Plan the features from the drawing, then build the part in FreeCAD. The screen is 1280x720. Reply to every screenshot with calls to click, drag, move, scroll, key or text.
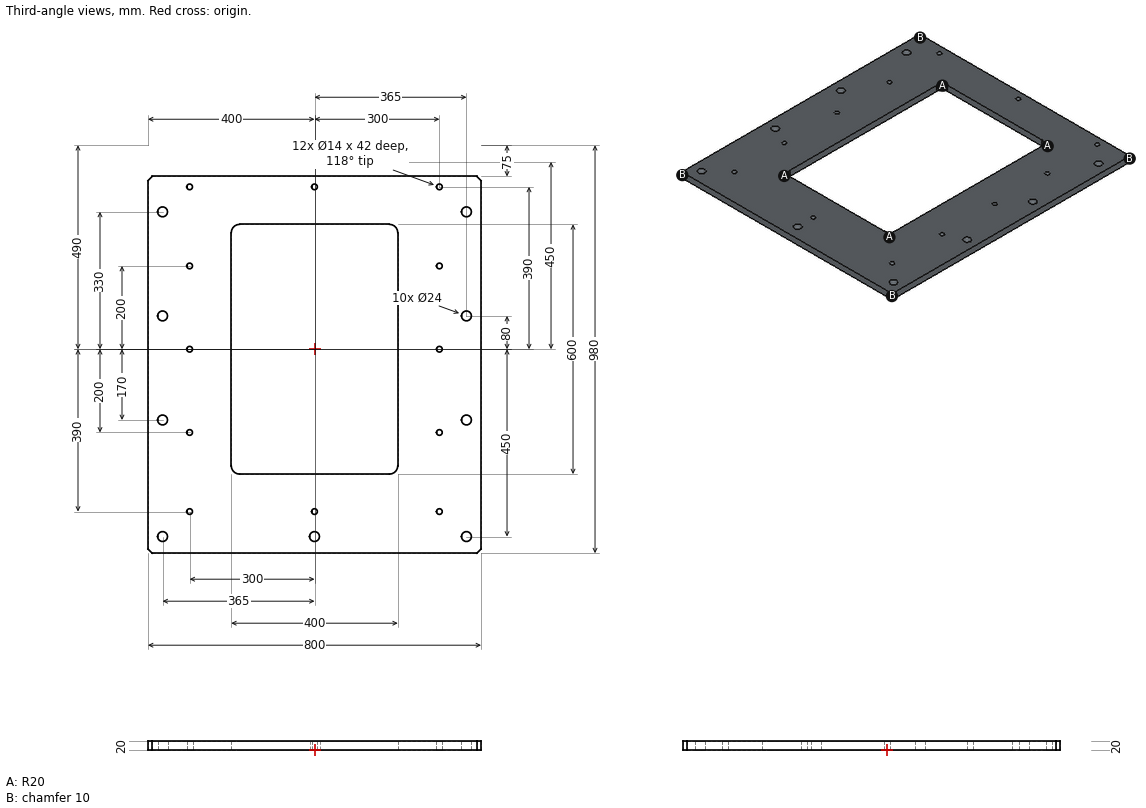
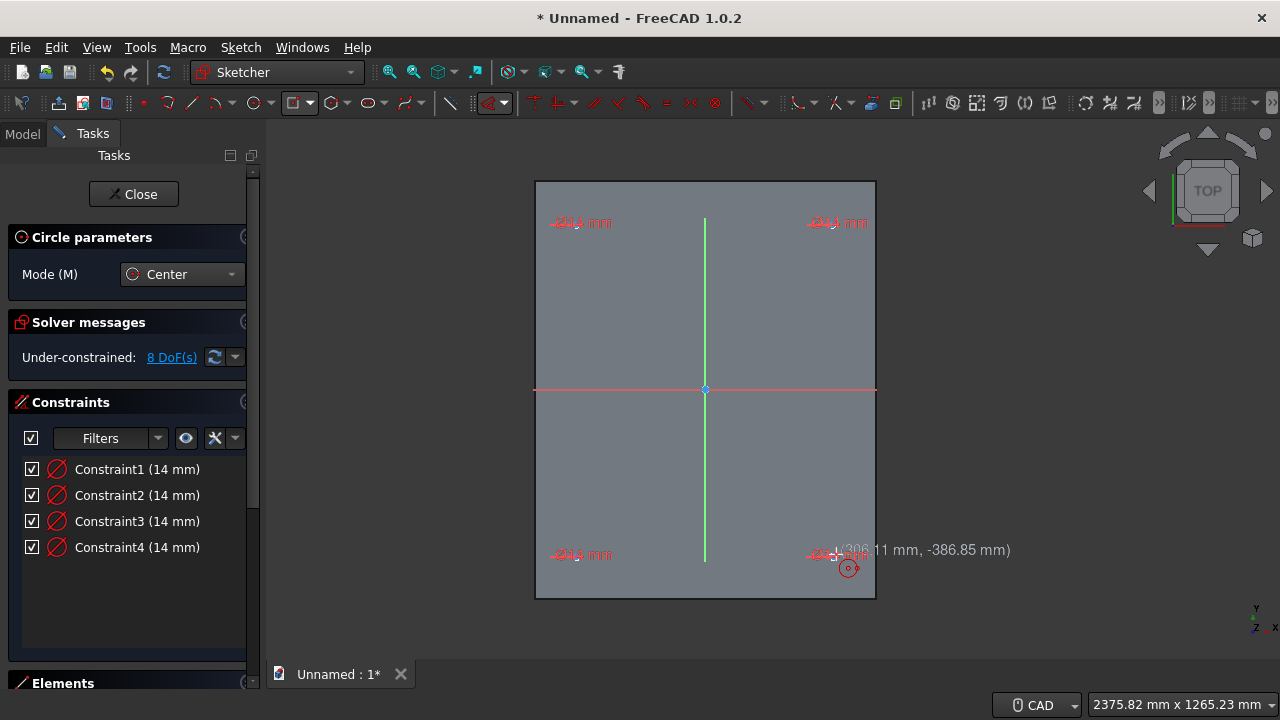
scroll(577, 390, up, 11)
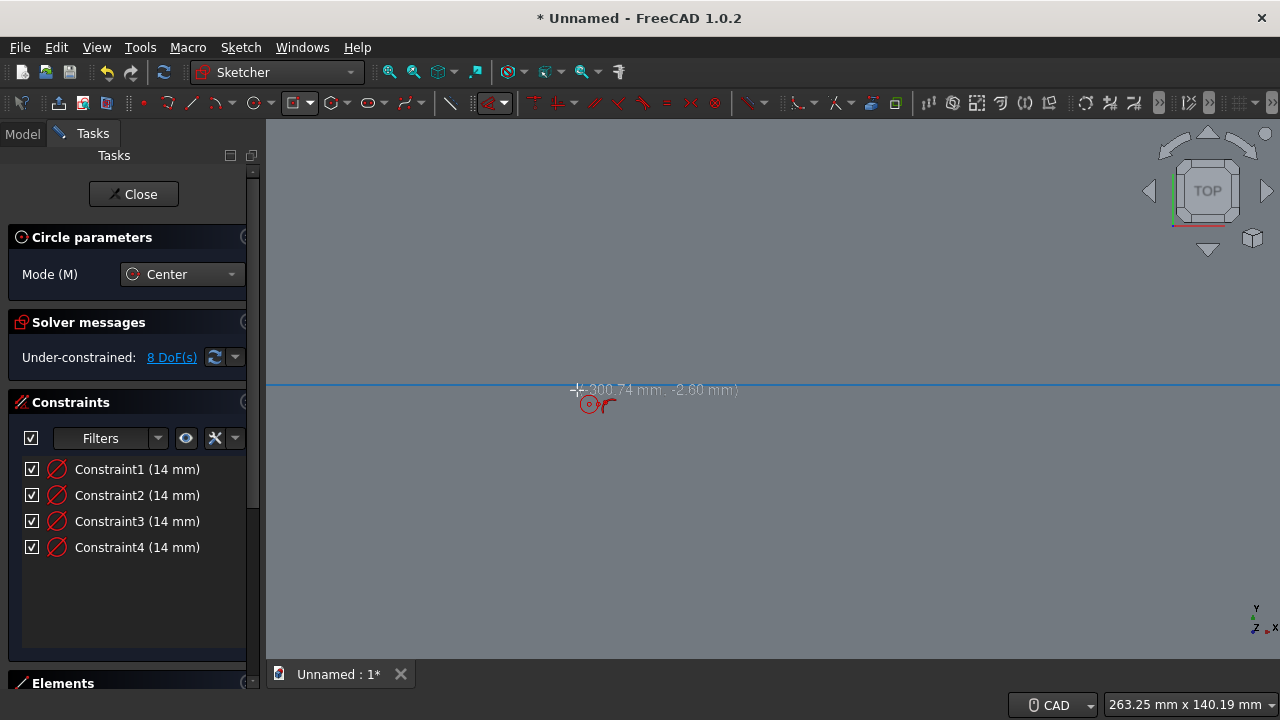
scroll(576, 390, down, 11)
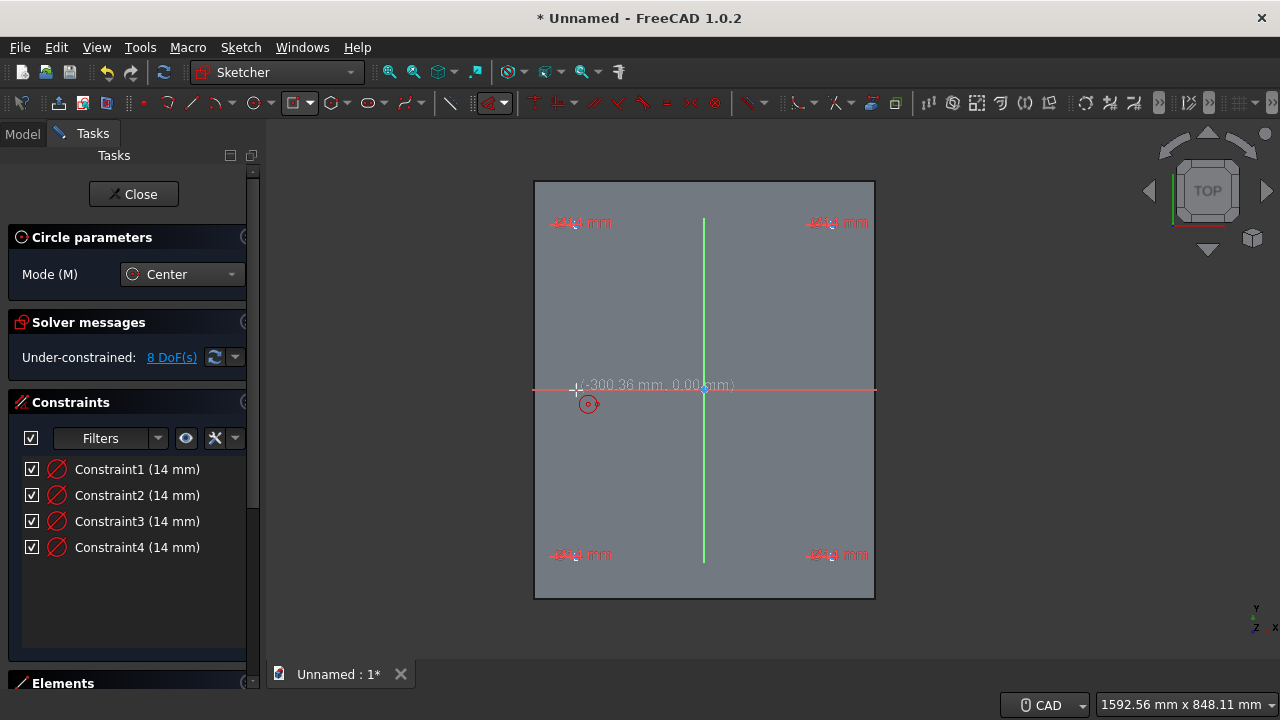
click(576, 390)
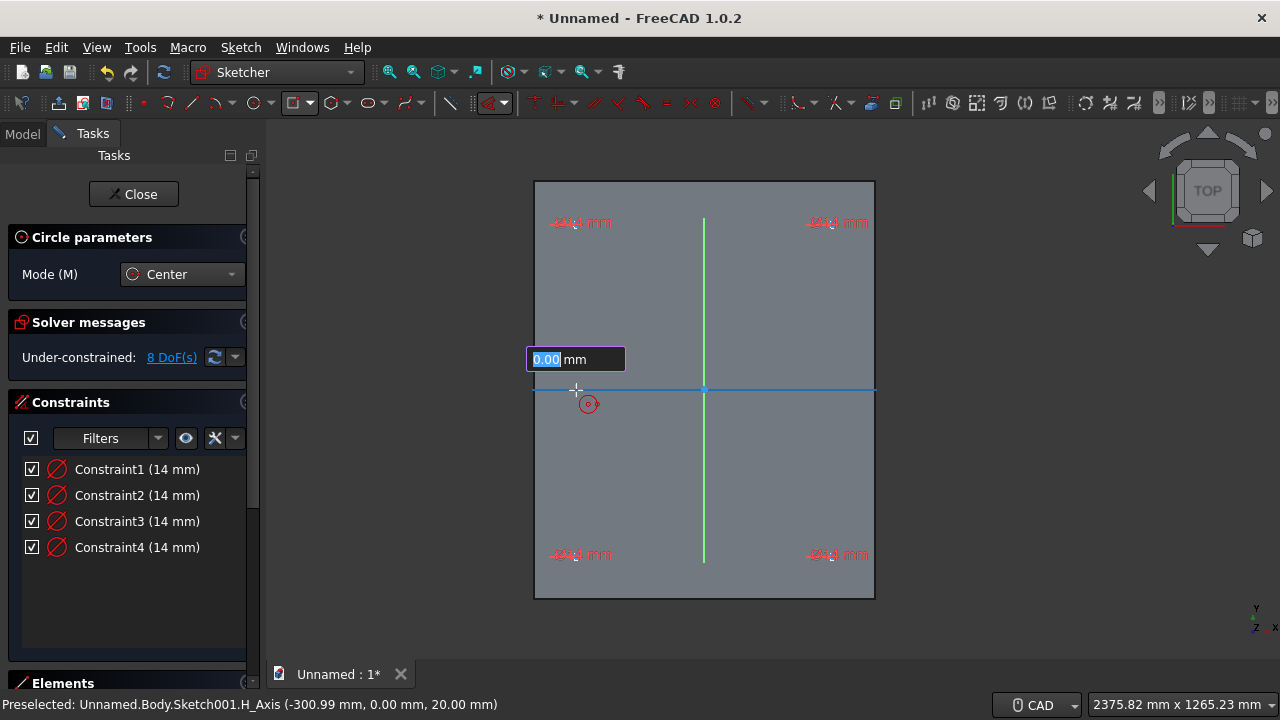
scroll(577, 387, up, 9)
move(578, 385)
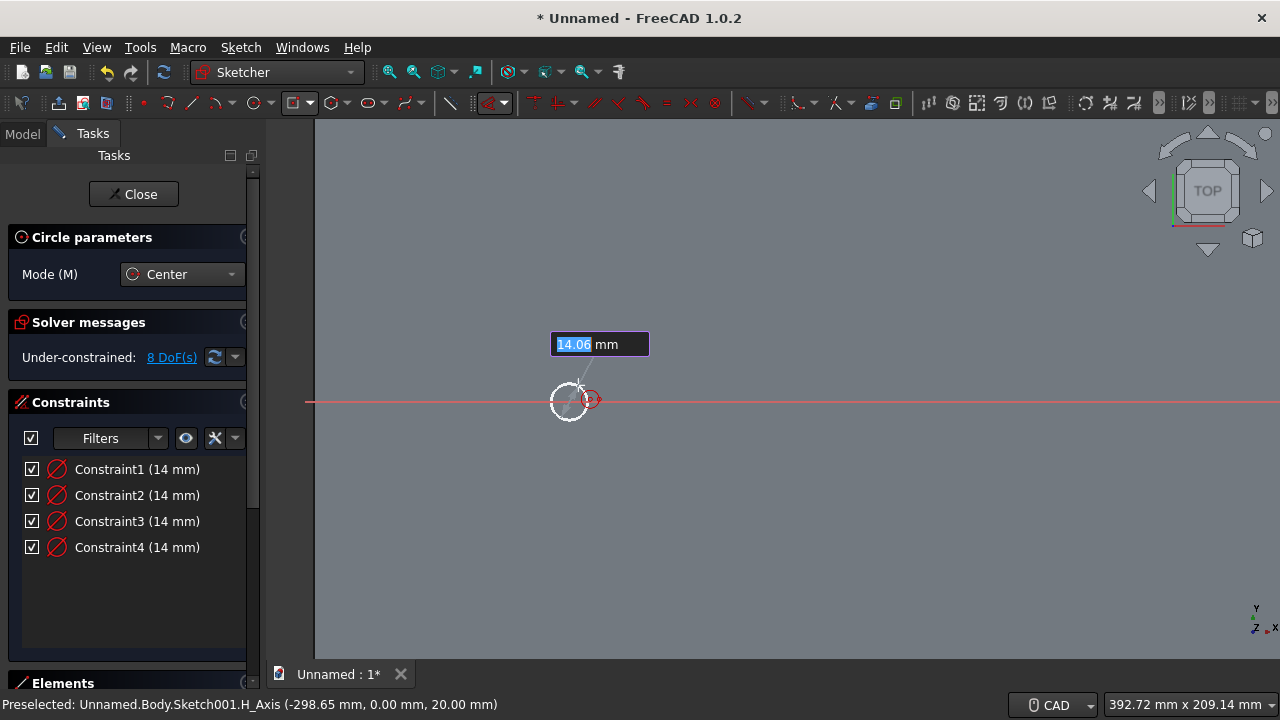
text(14)
key(Return)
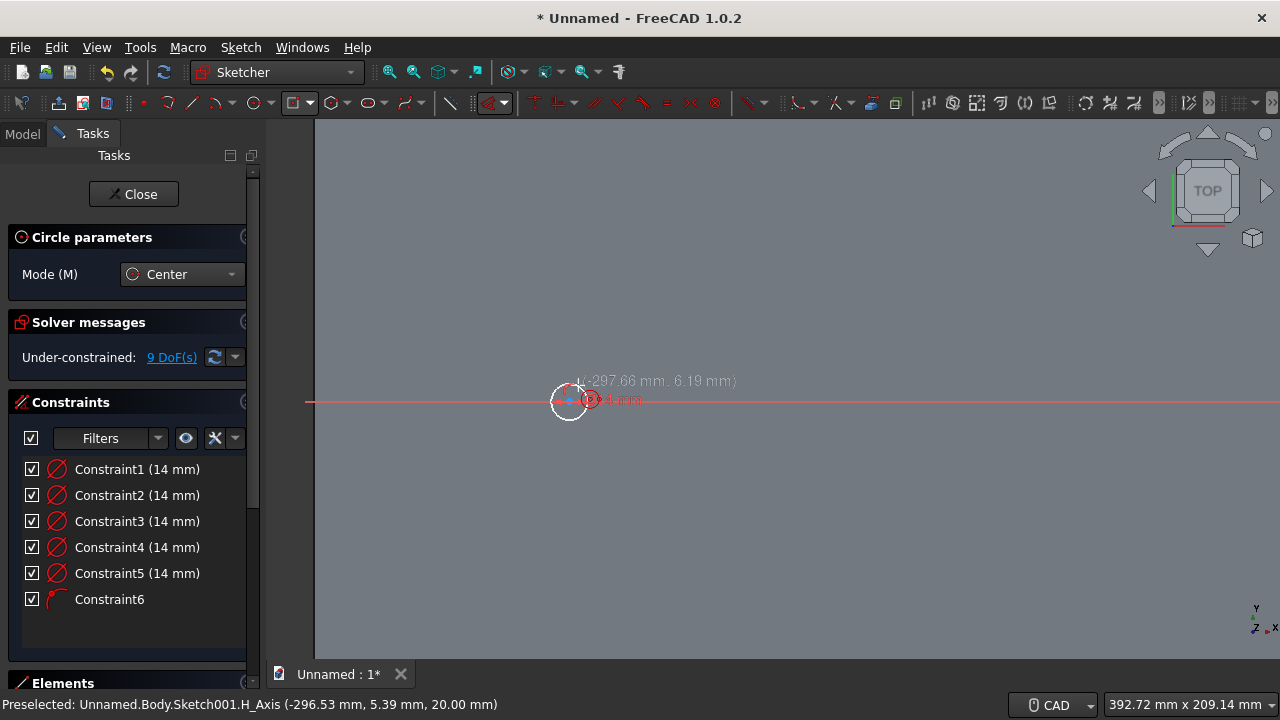
scroll(577, 386, down, 9)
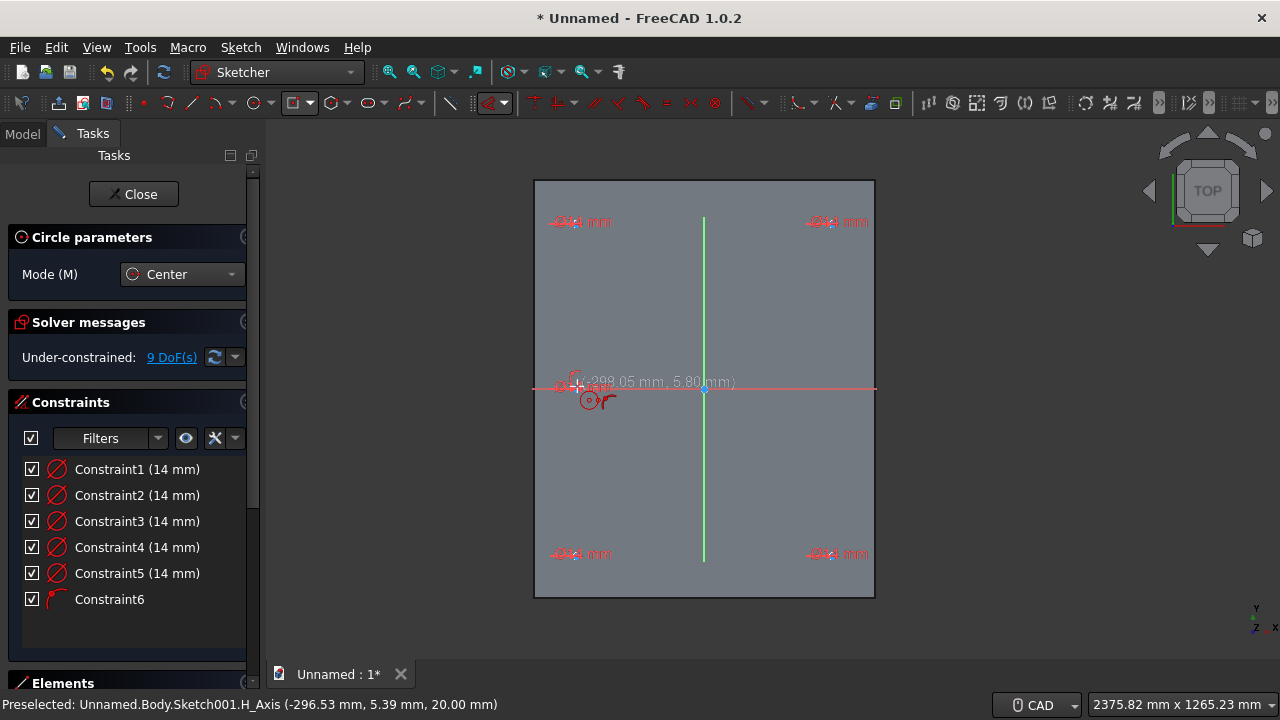
scroll(704, 556, up, 11)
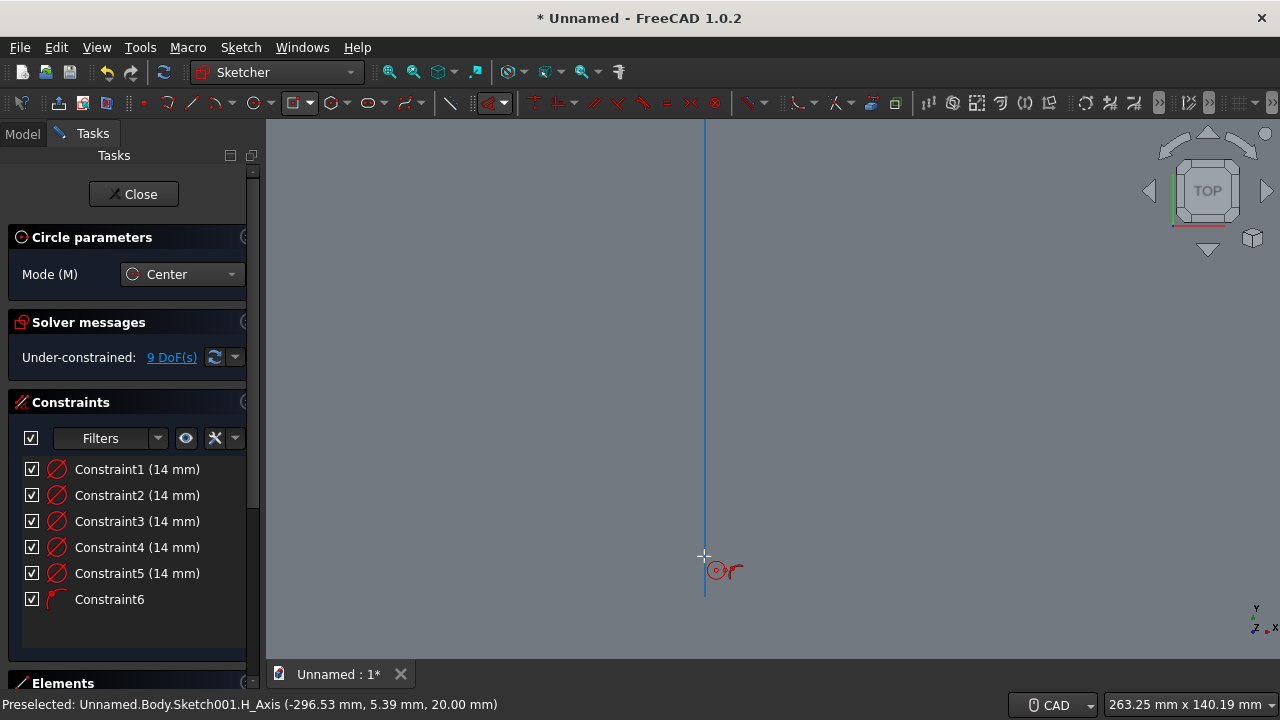
scroll(704, 557, down, 11)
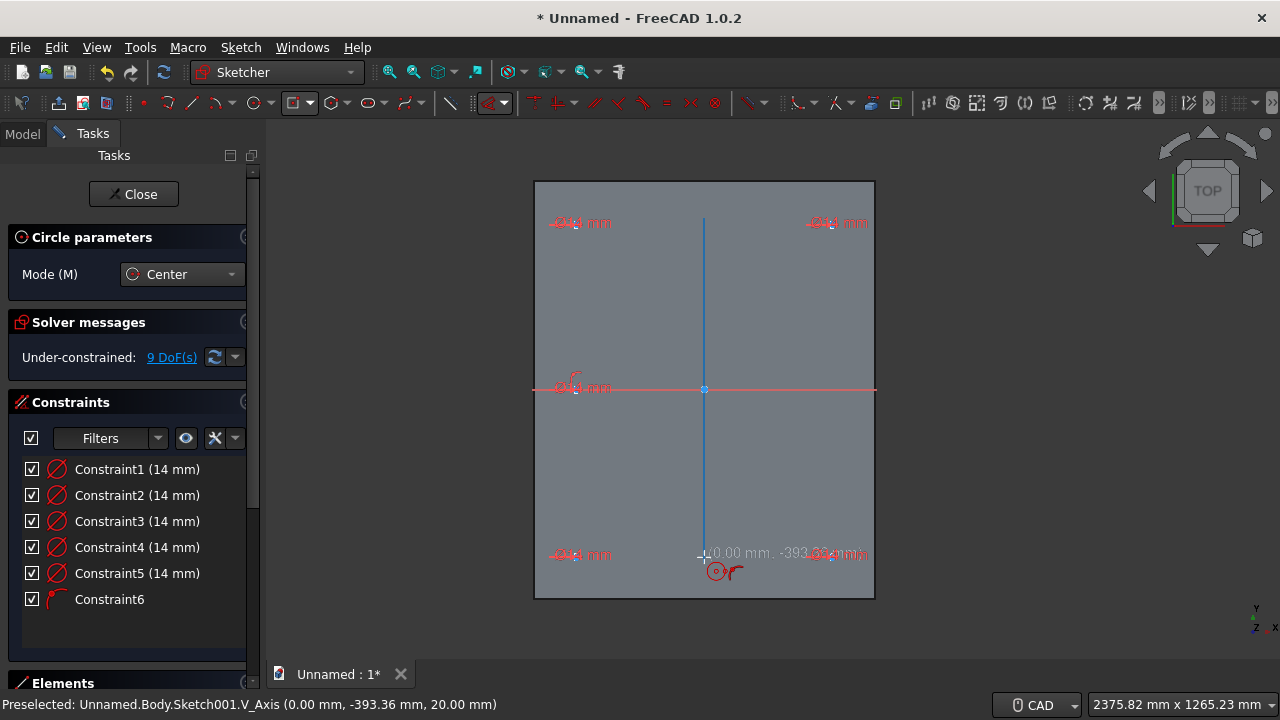
click(704, 556)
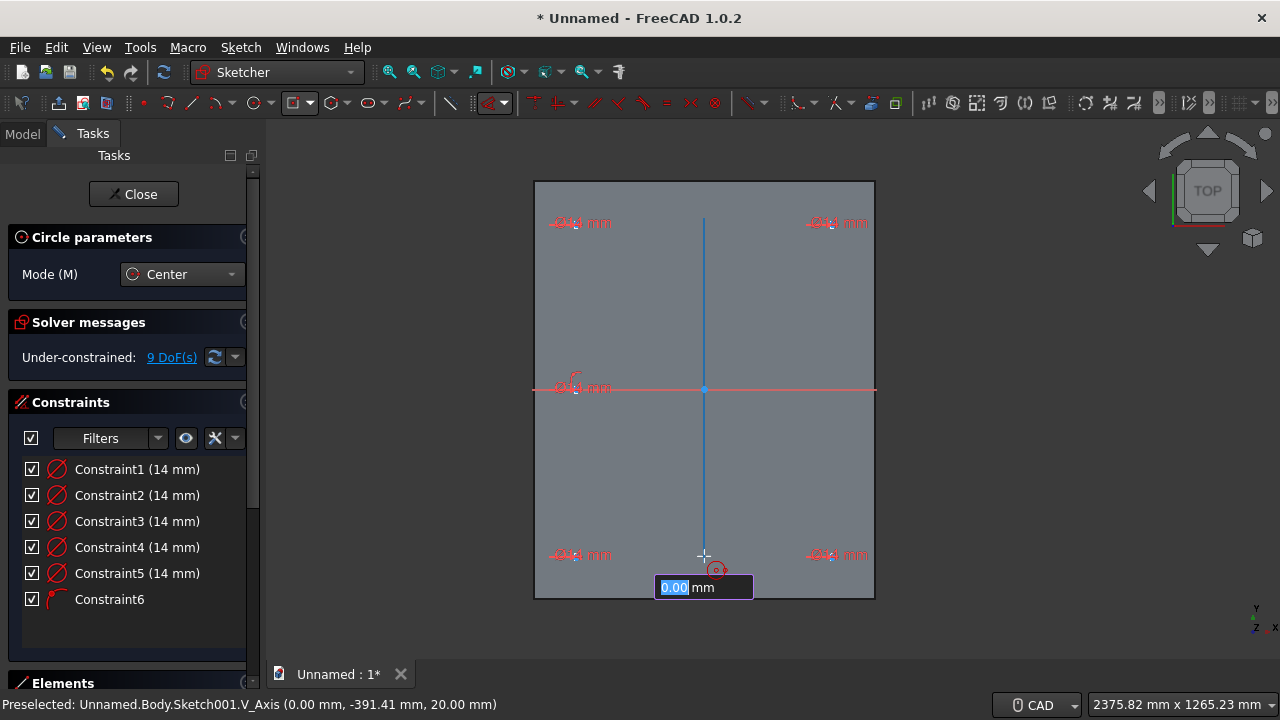
scroll(707, 555, up, 9)
move(706, 553)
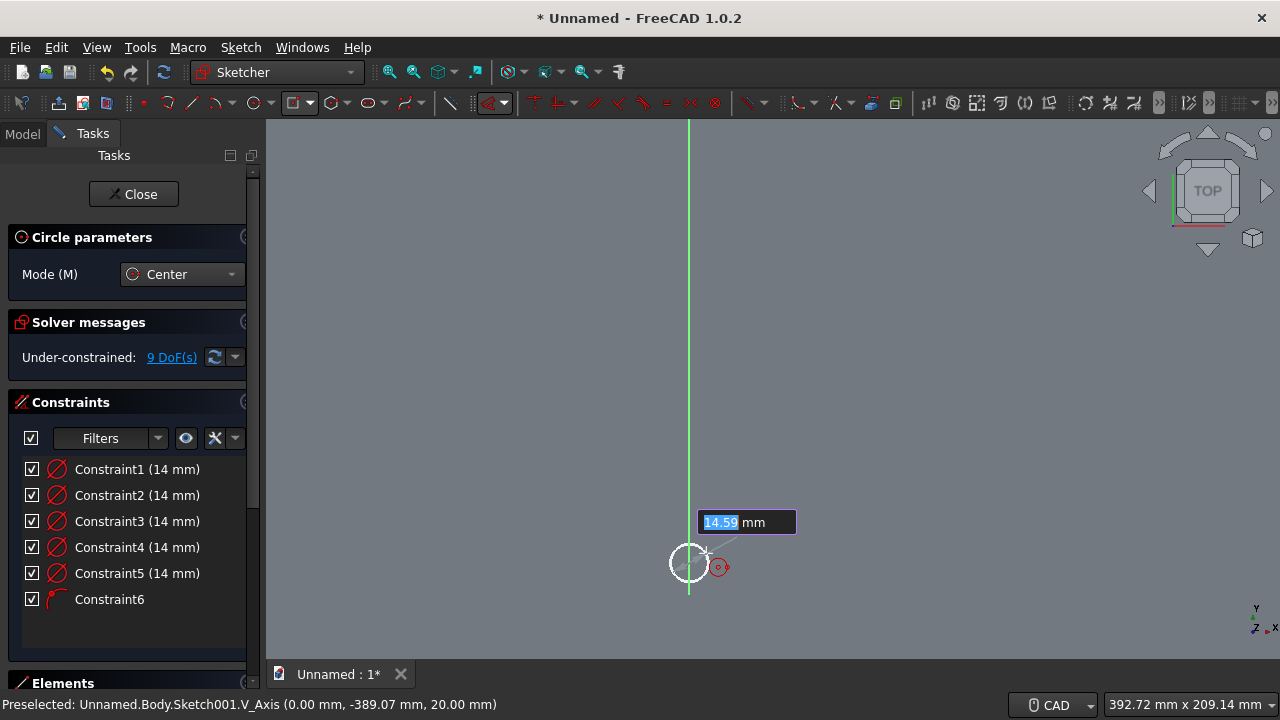
text(14)
key(Return)